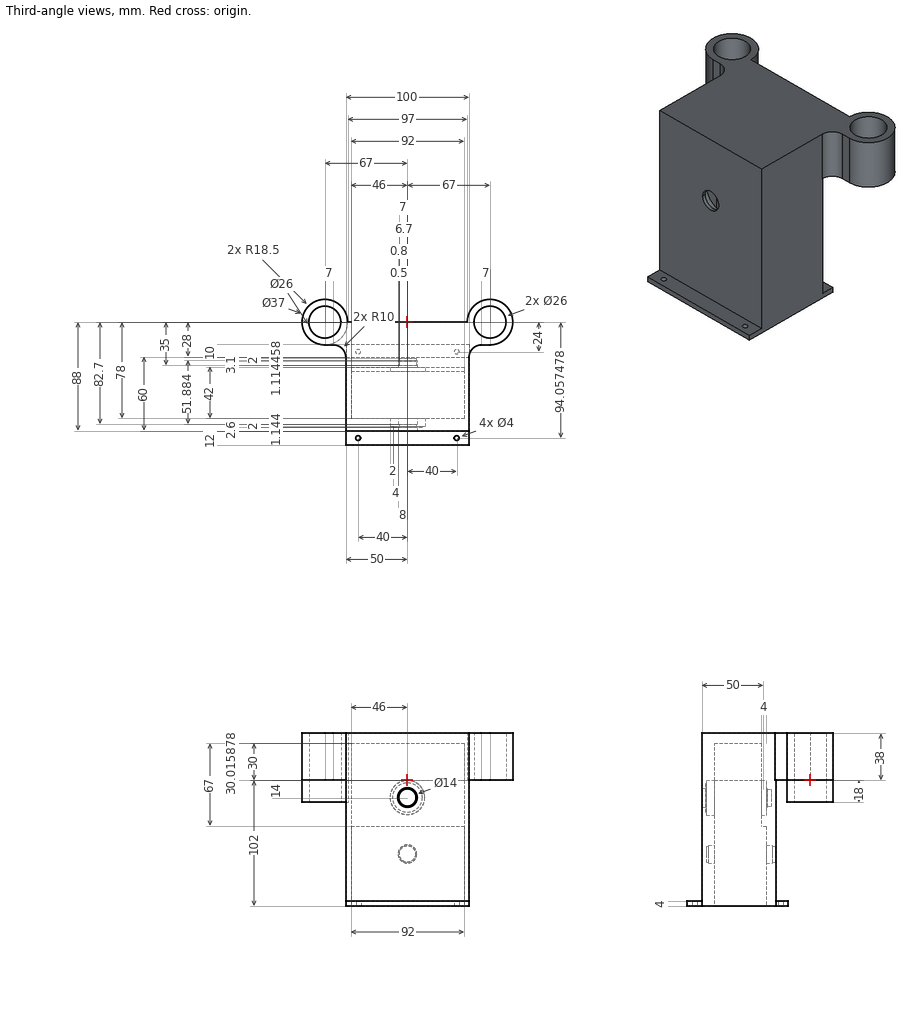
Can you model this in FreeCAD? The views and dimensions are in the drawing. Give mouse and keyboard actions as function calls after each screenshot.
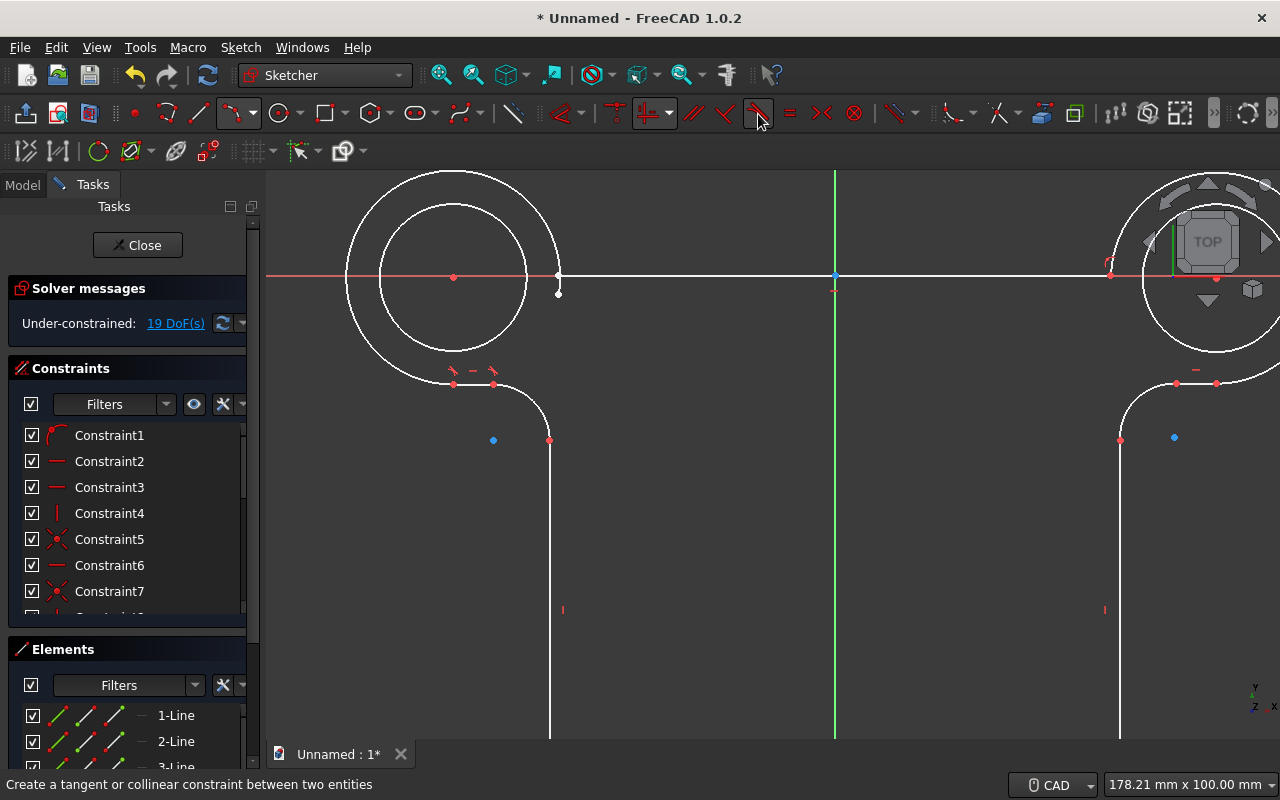
click(550, 542)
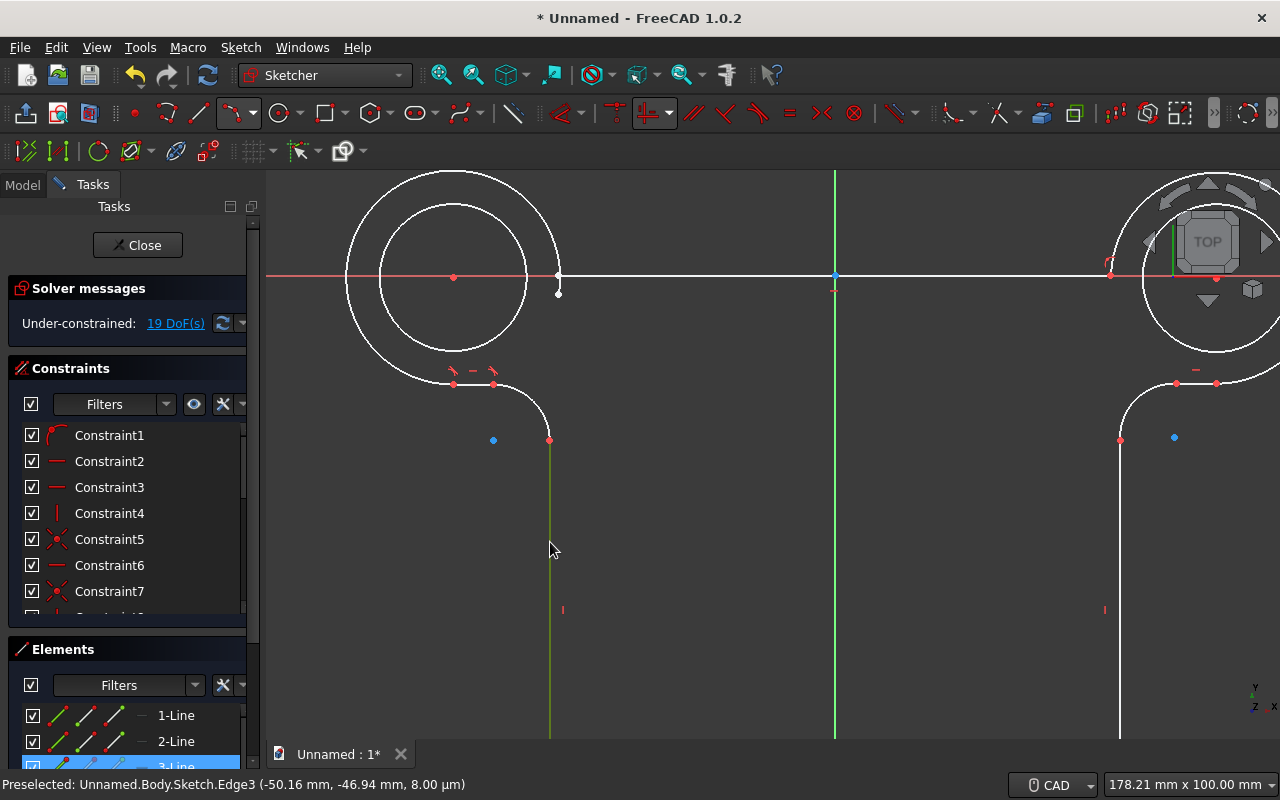
click(543, 415)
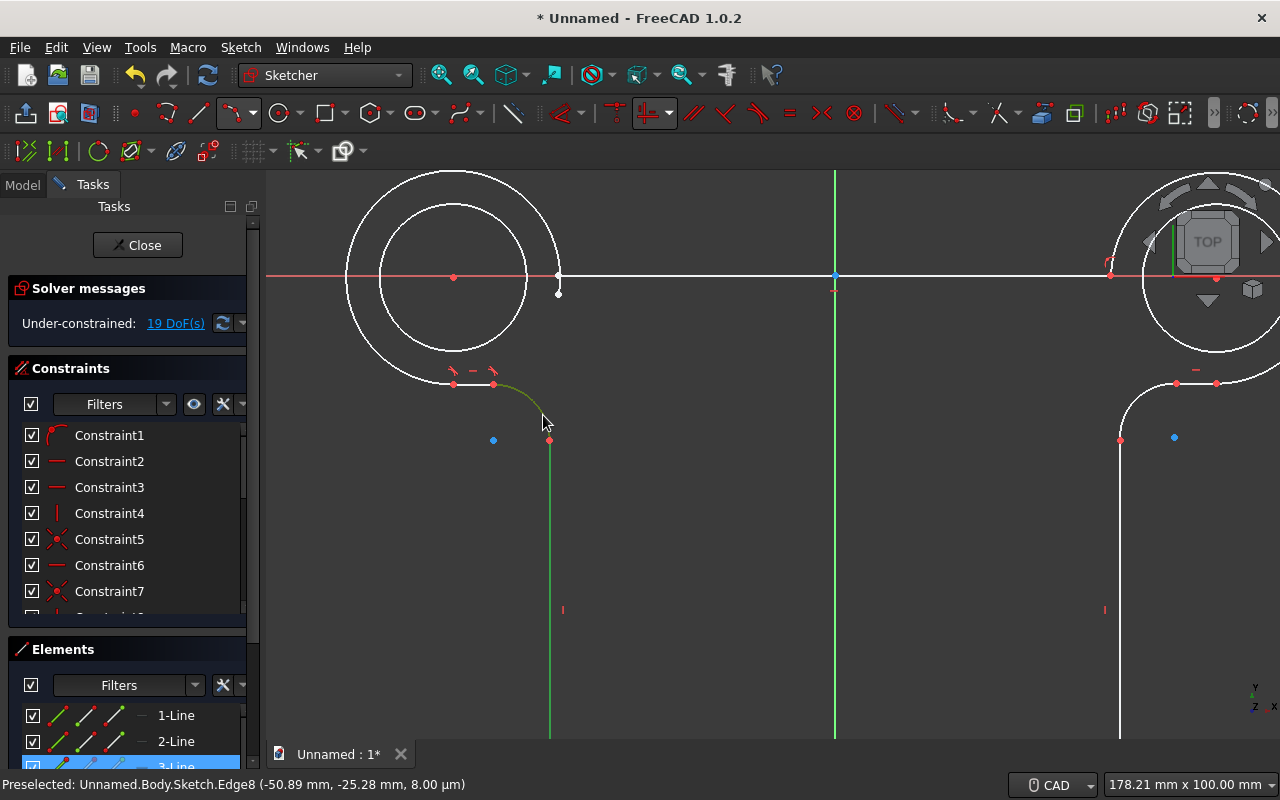
key(t)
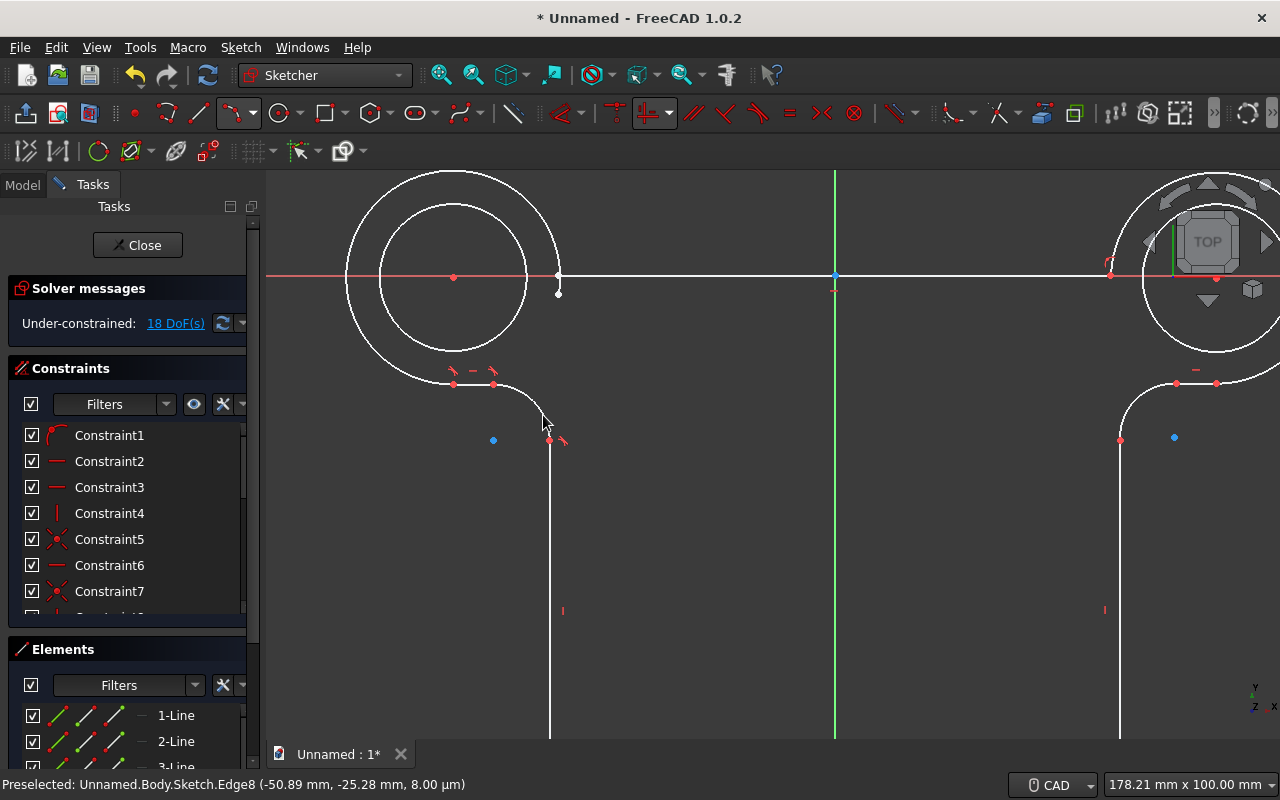
scroll(439, 384, down, 2)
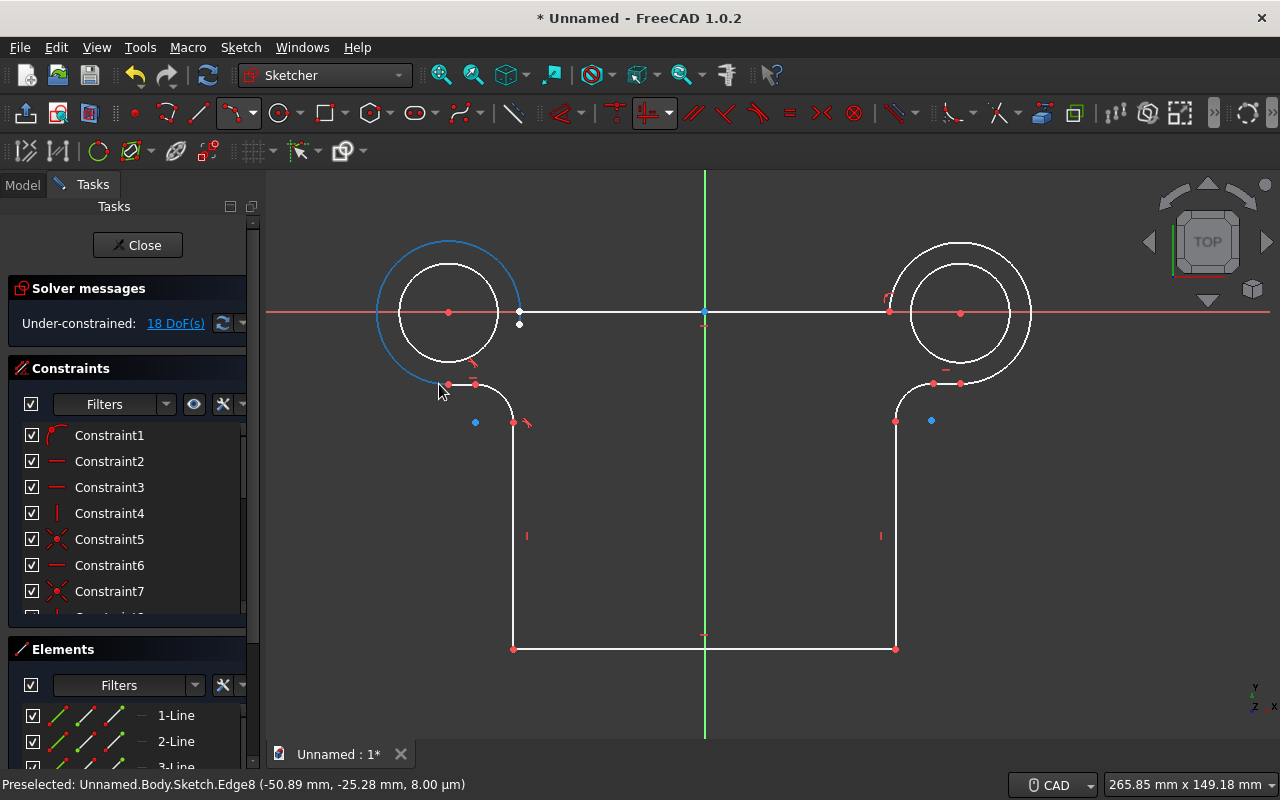
click(896, 581)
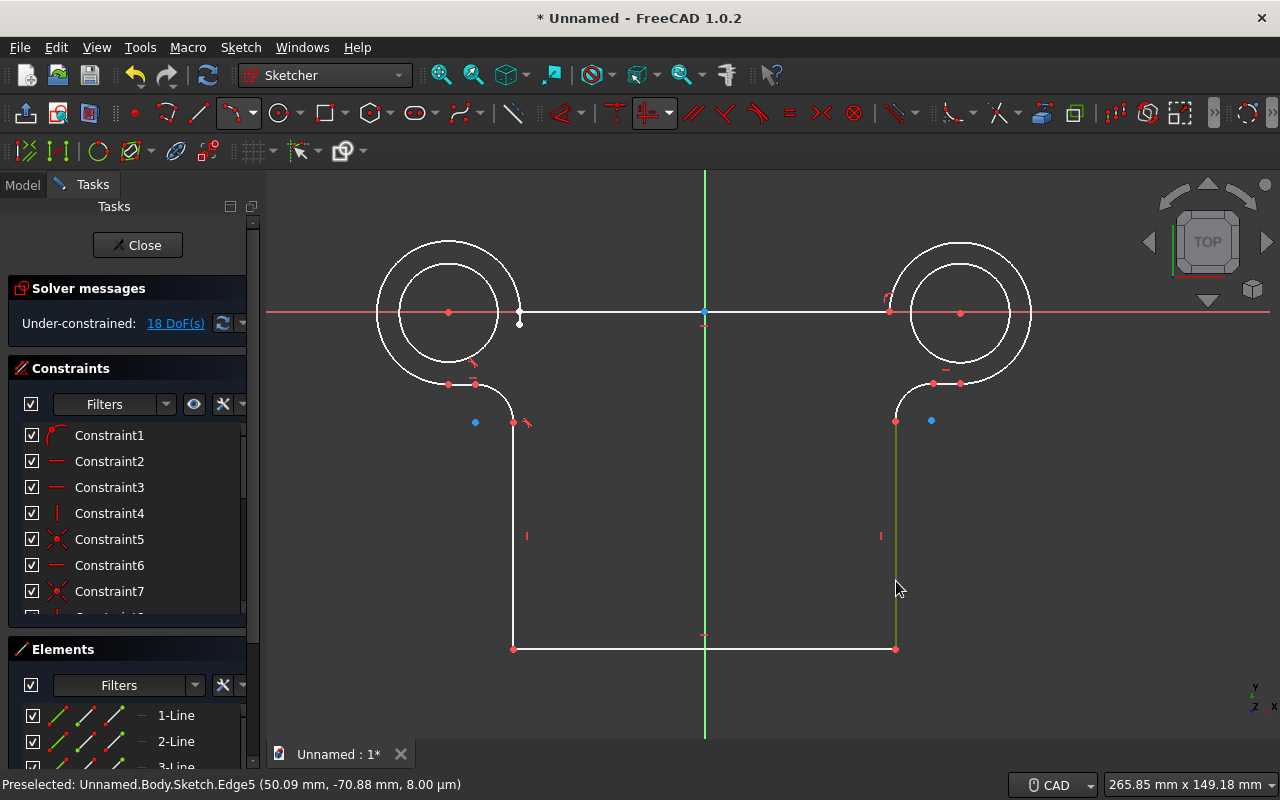
click(916, 388)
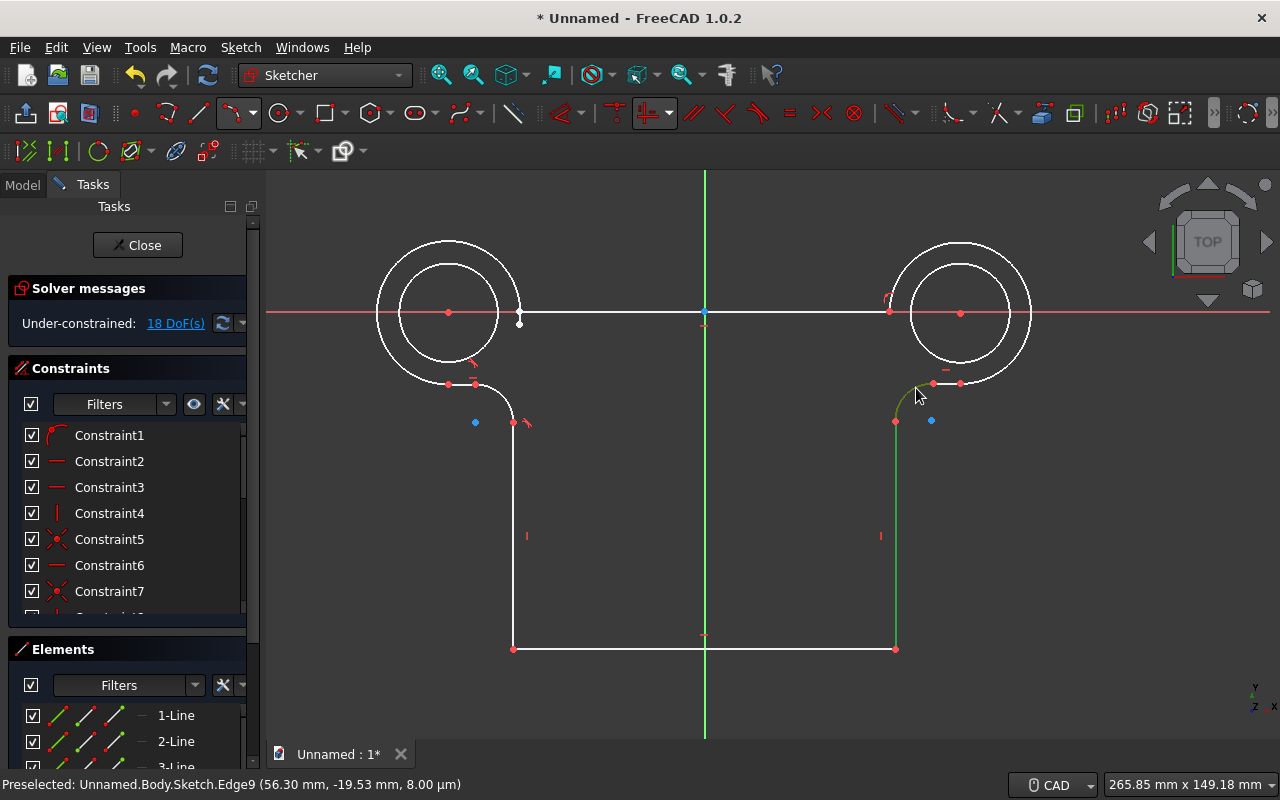
key(t)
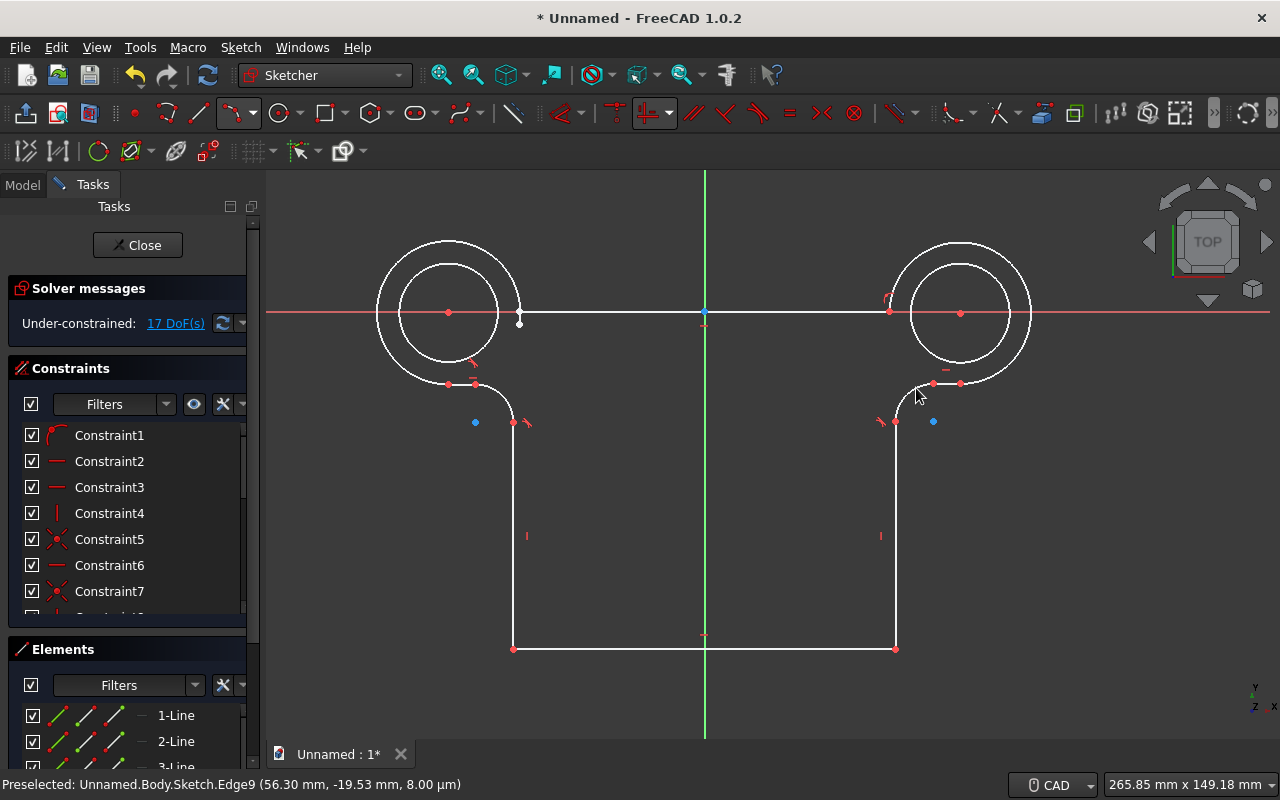
scroll(944, 384, up, 2)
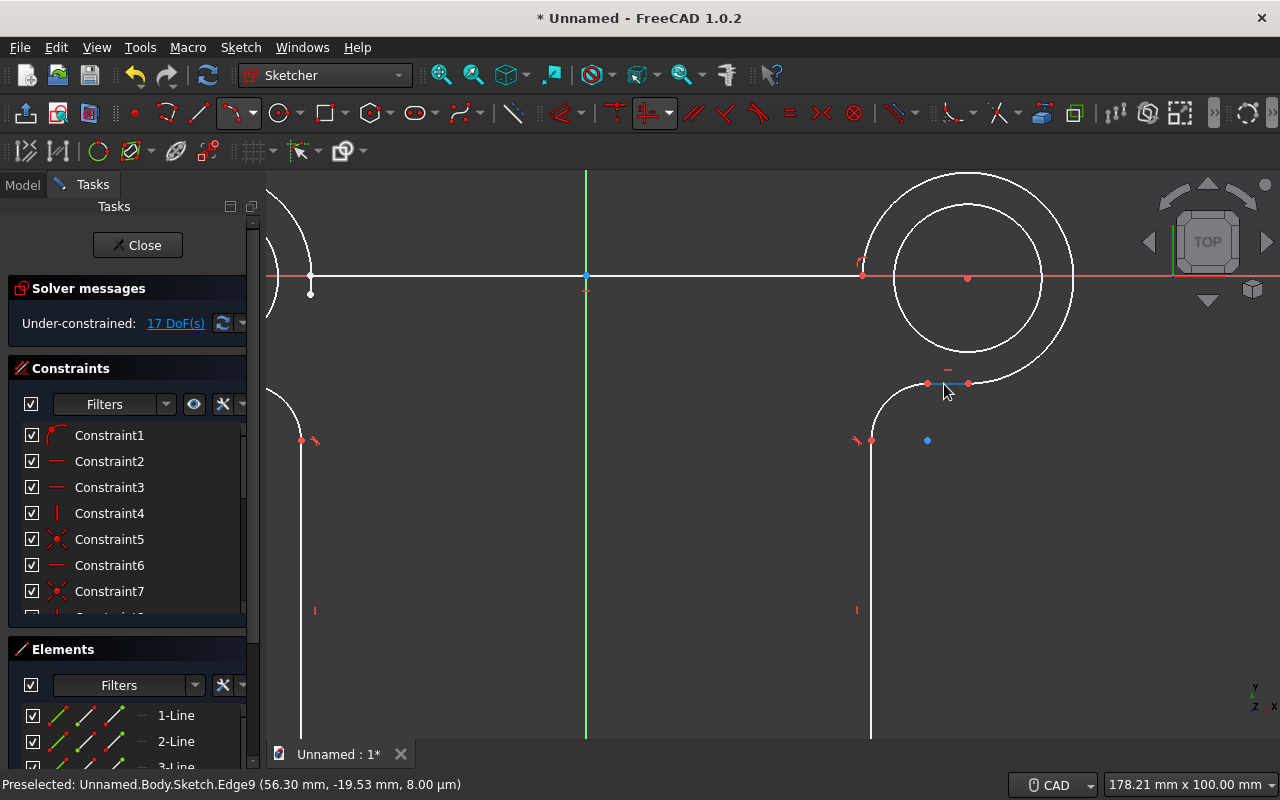
click(944, 384)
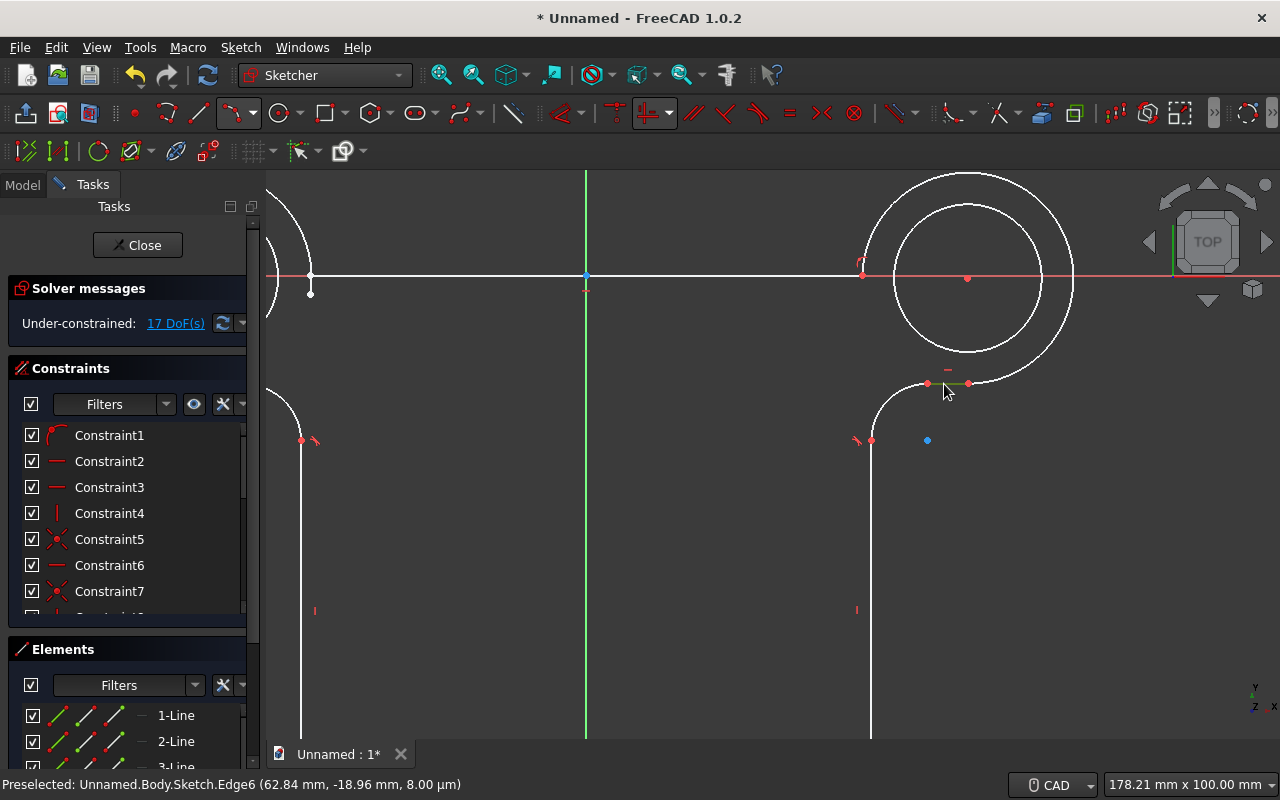
click(902, 390)